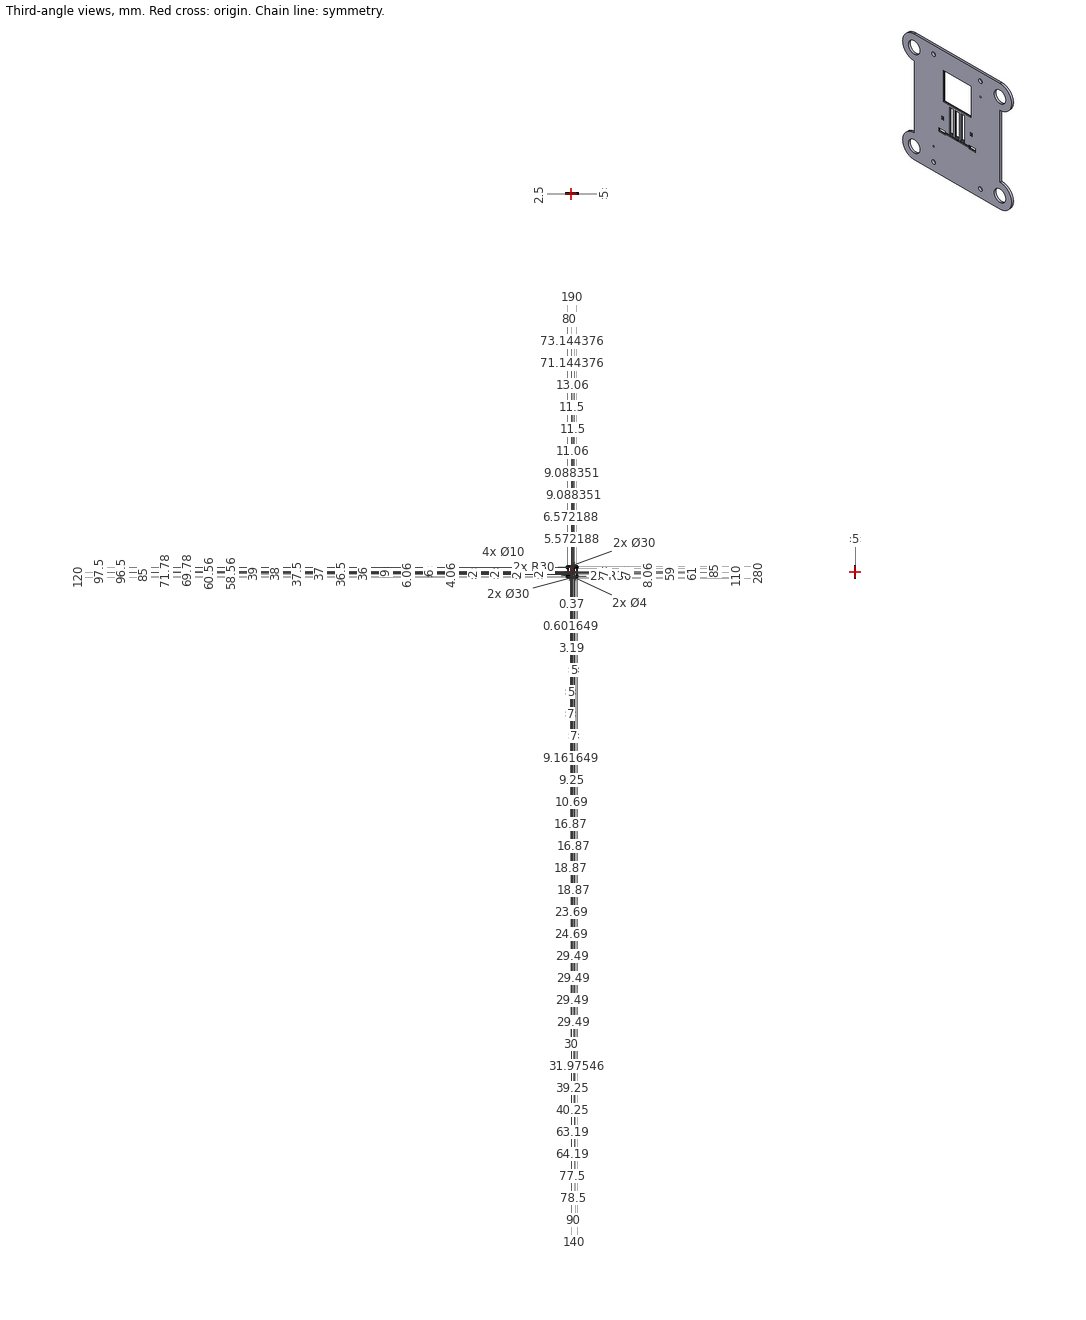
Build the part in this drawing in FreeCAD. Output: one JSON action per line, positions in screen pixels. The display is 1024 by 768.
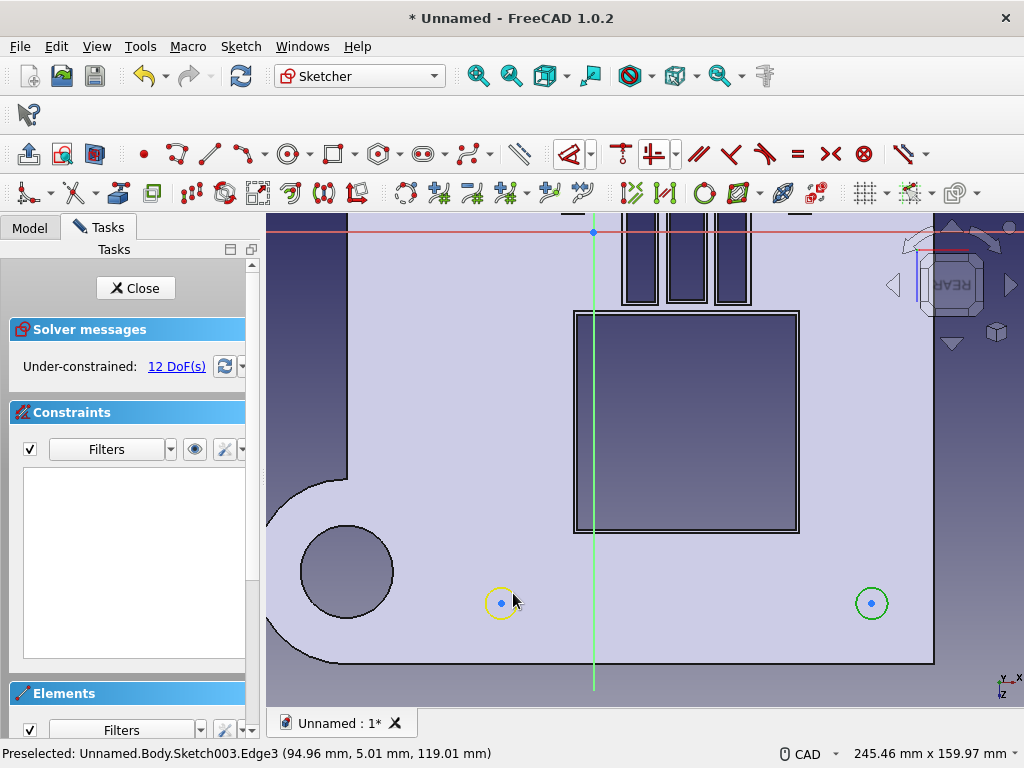
{"action": "left_click", "coordinate": [512, 592]}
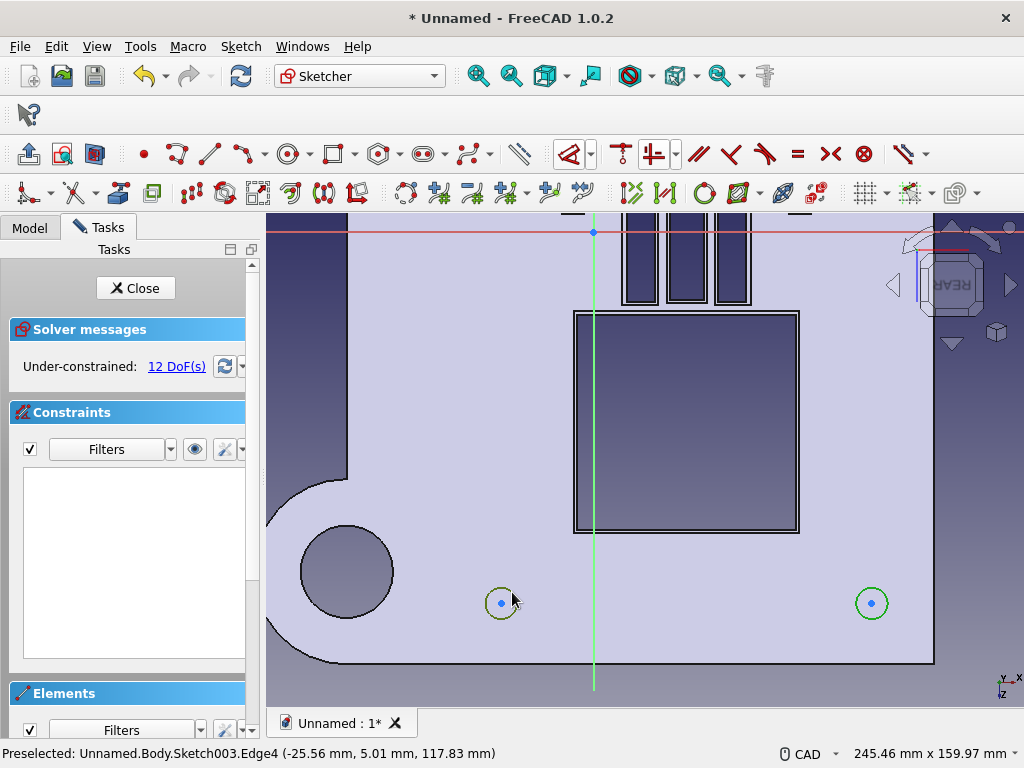
{"action": "left_click", "coordinate": [798, 154]}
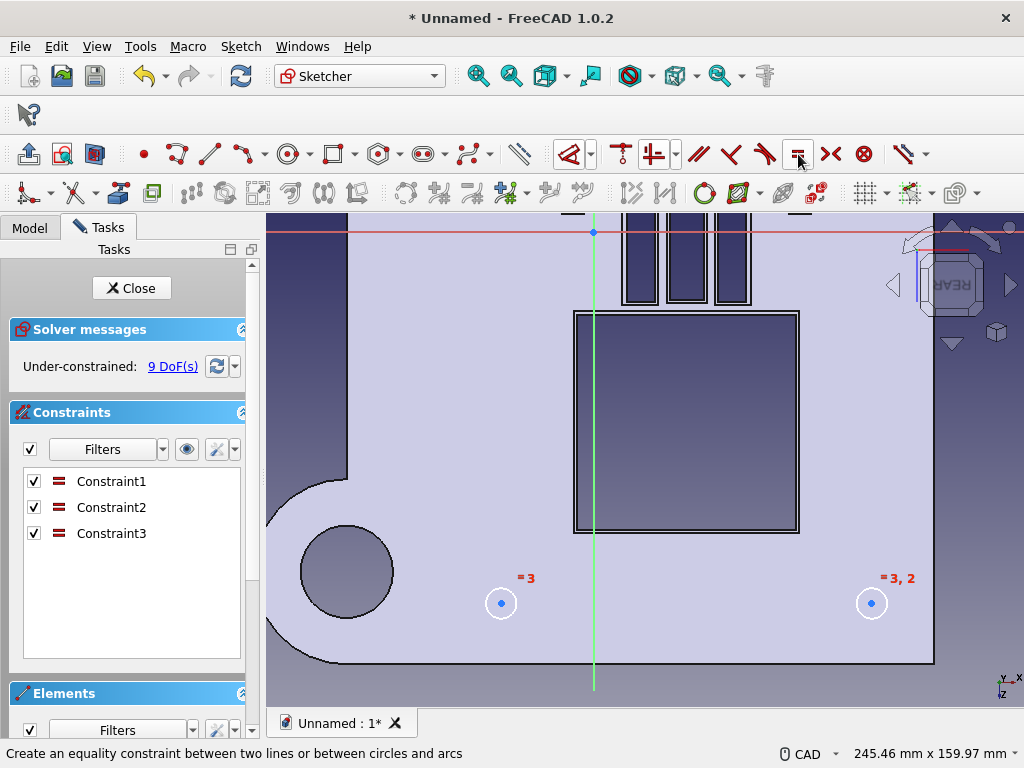
{"action": "scroll", "coordinate": [512, 593], "scroll_direction": "down", "scroll_amount": 5}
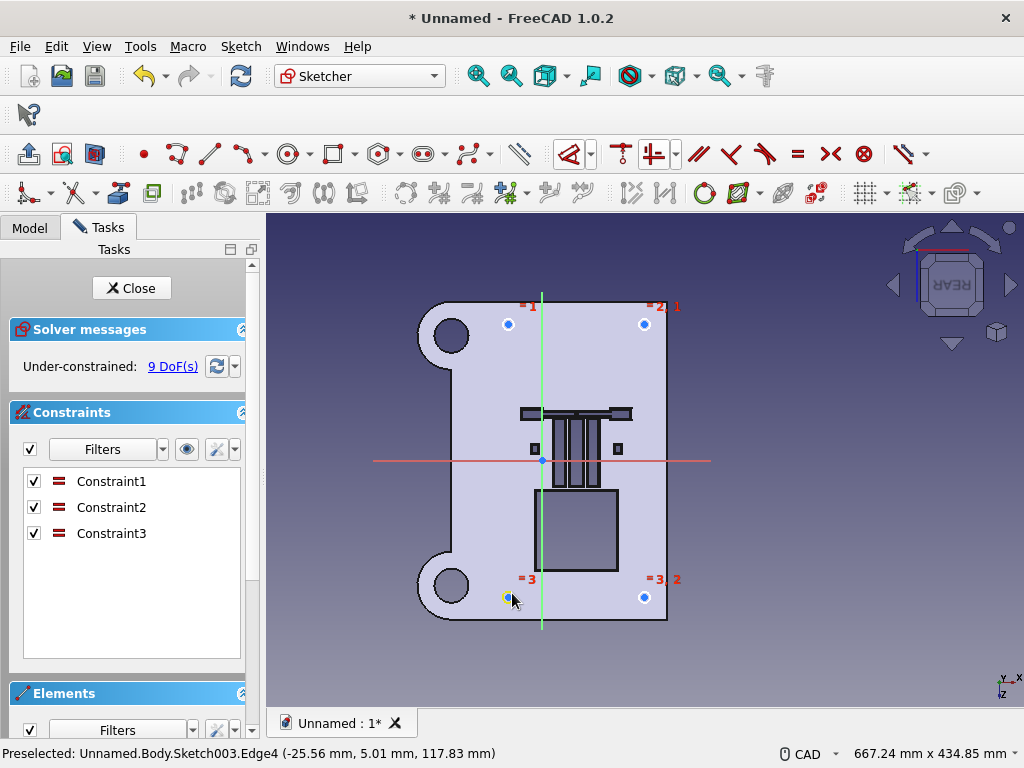
{"action": "left_click", "coordinate": [645, 325]}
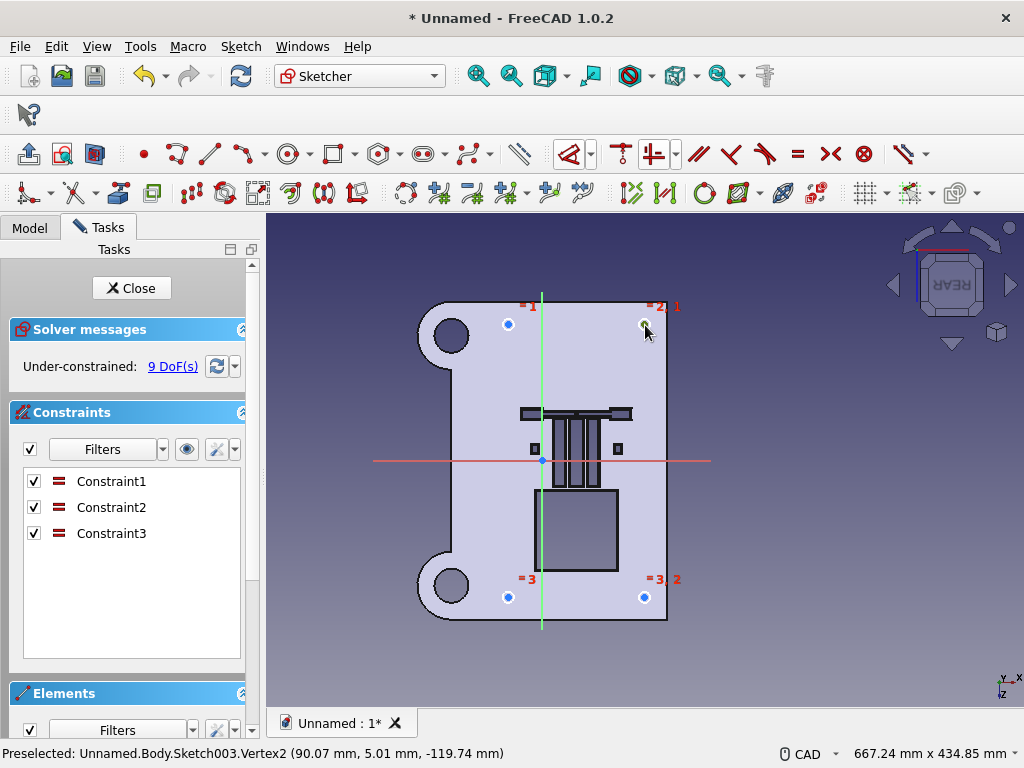
{"action": "left_click", "coordinate": [645, 597]}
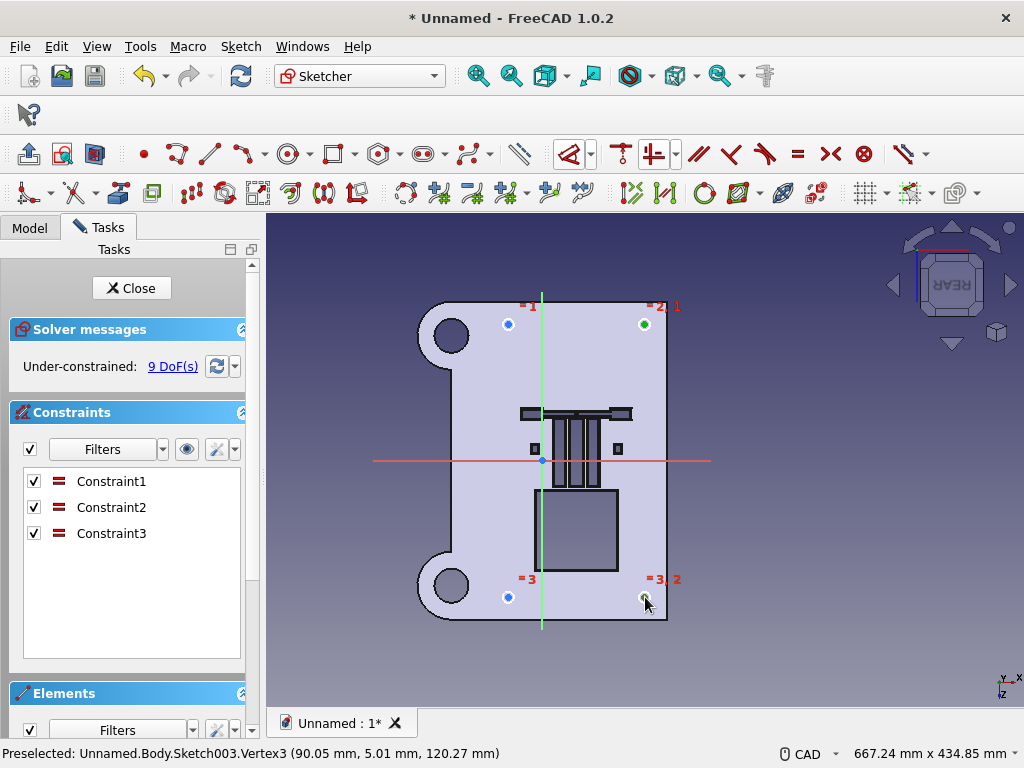
{"action": "left_click", "coordinate": [375, 461]}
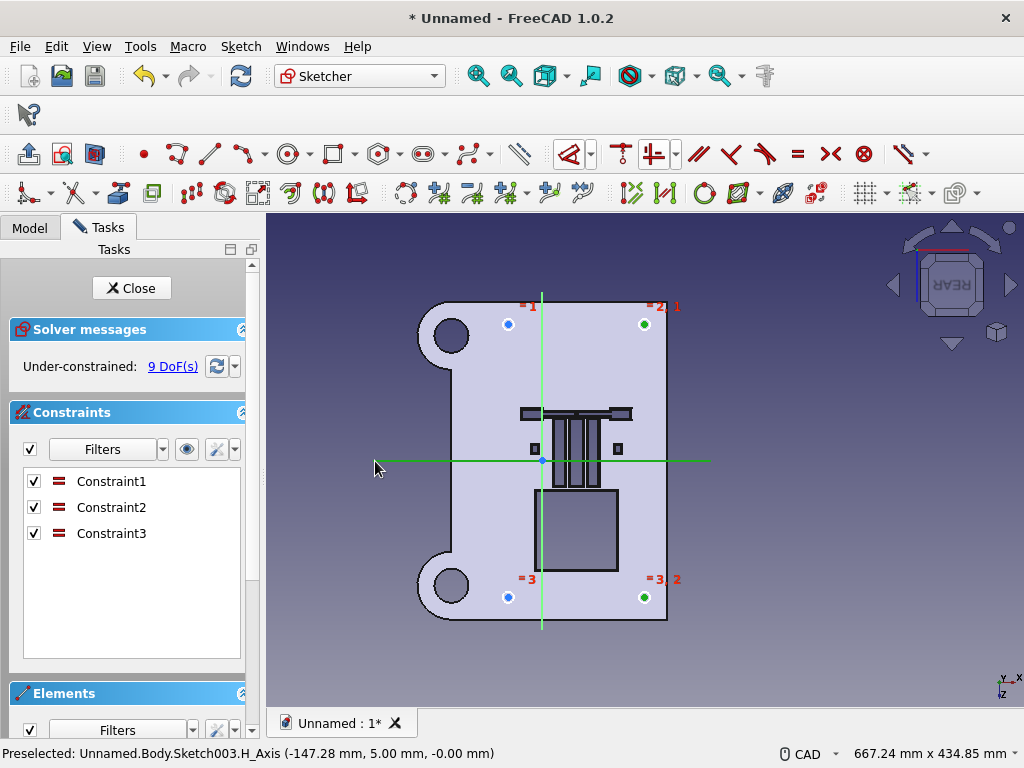
{"action": "left_click", "coordinate": [831, 154]}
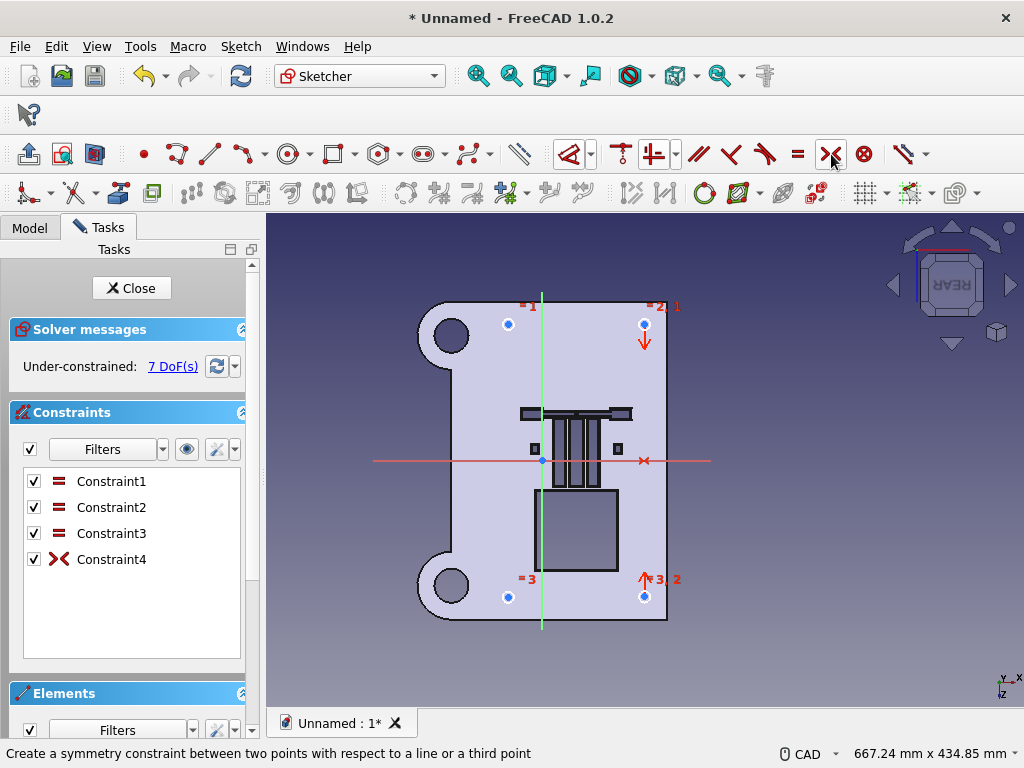
{"action": "left_click", "coordinate": [508, 325]}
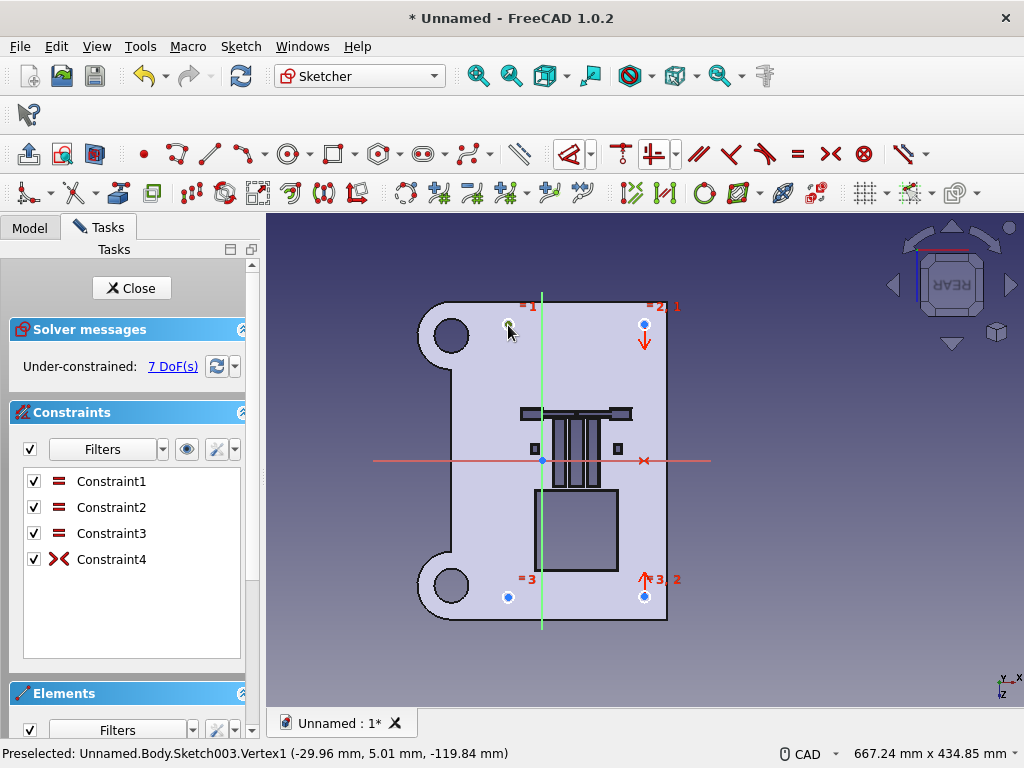
{"action": "left_click", "coordinate": [508, 597]}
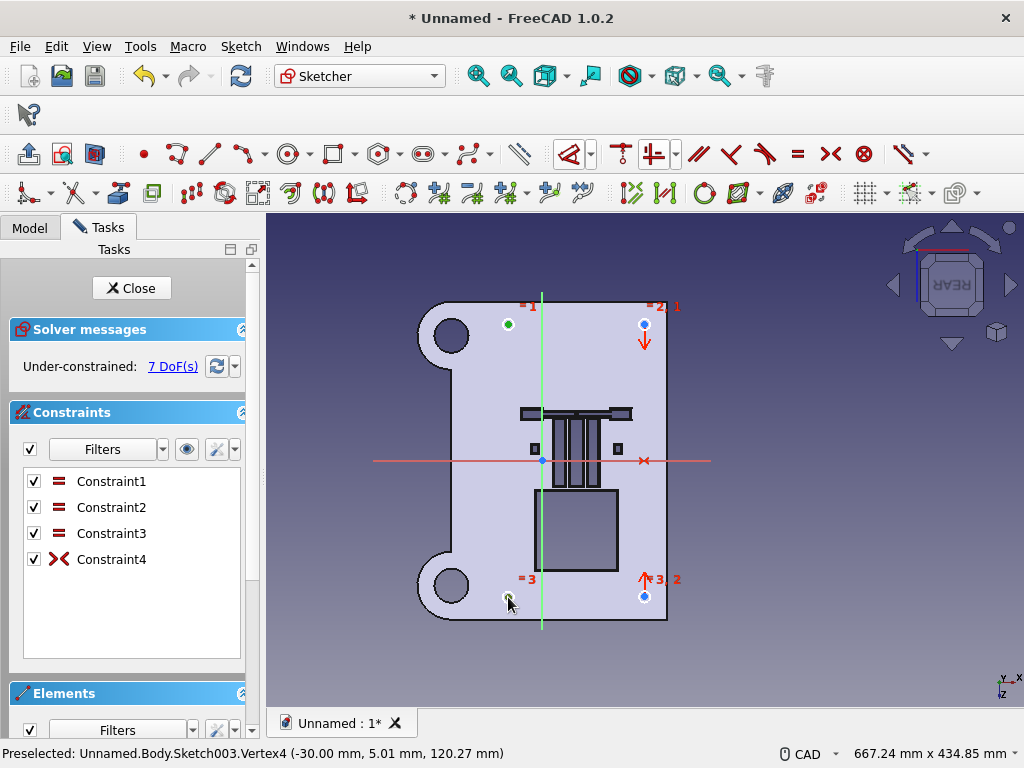
{"action": "left_click", "coordinate": [375, 461]}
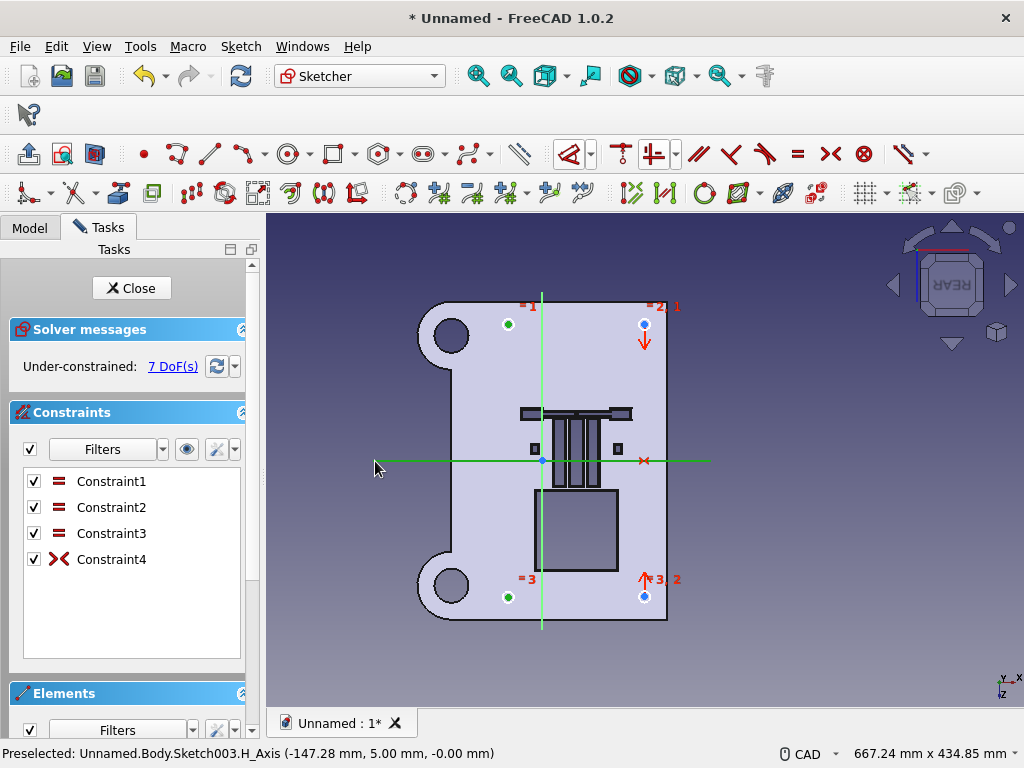
{"action": "left_click", "coordinate": [831, 154]}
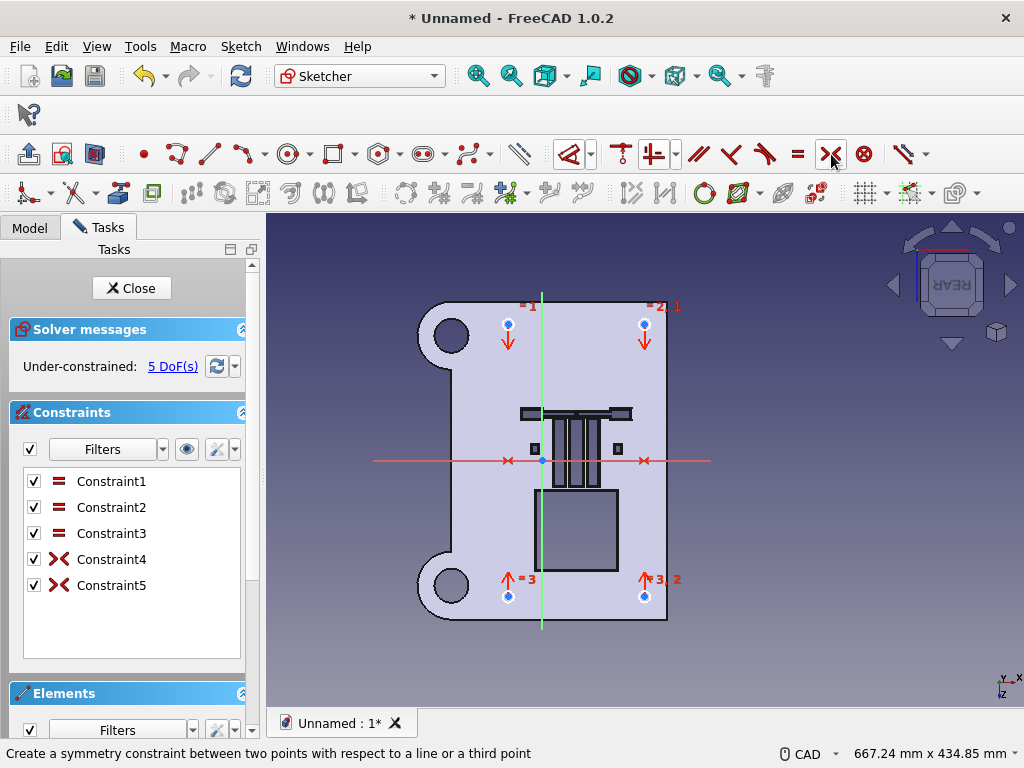
{"action": "scroll", "coordinate": [508, 319], "scroll_direction": "up", "scroll_amount": 7}